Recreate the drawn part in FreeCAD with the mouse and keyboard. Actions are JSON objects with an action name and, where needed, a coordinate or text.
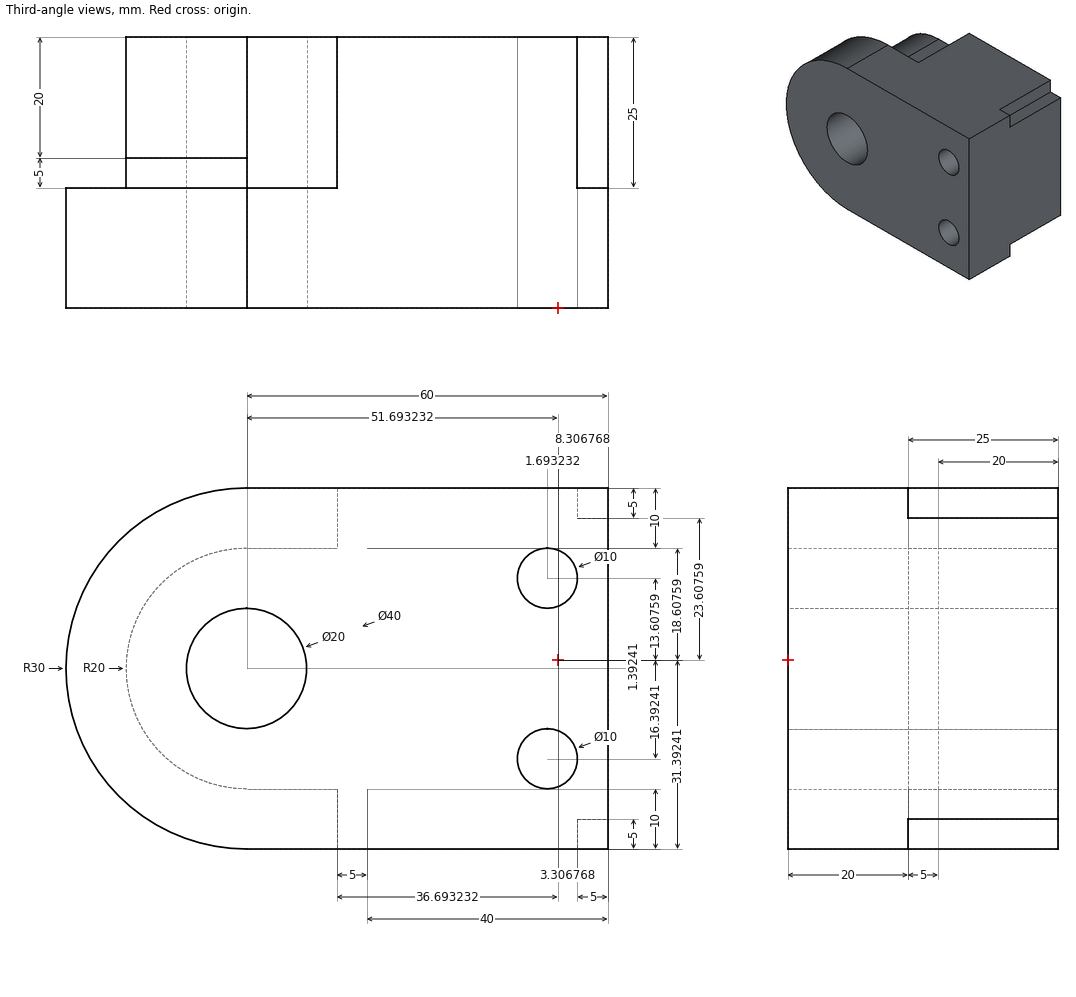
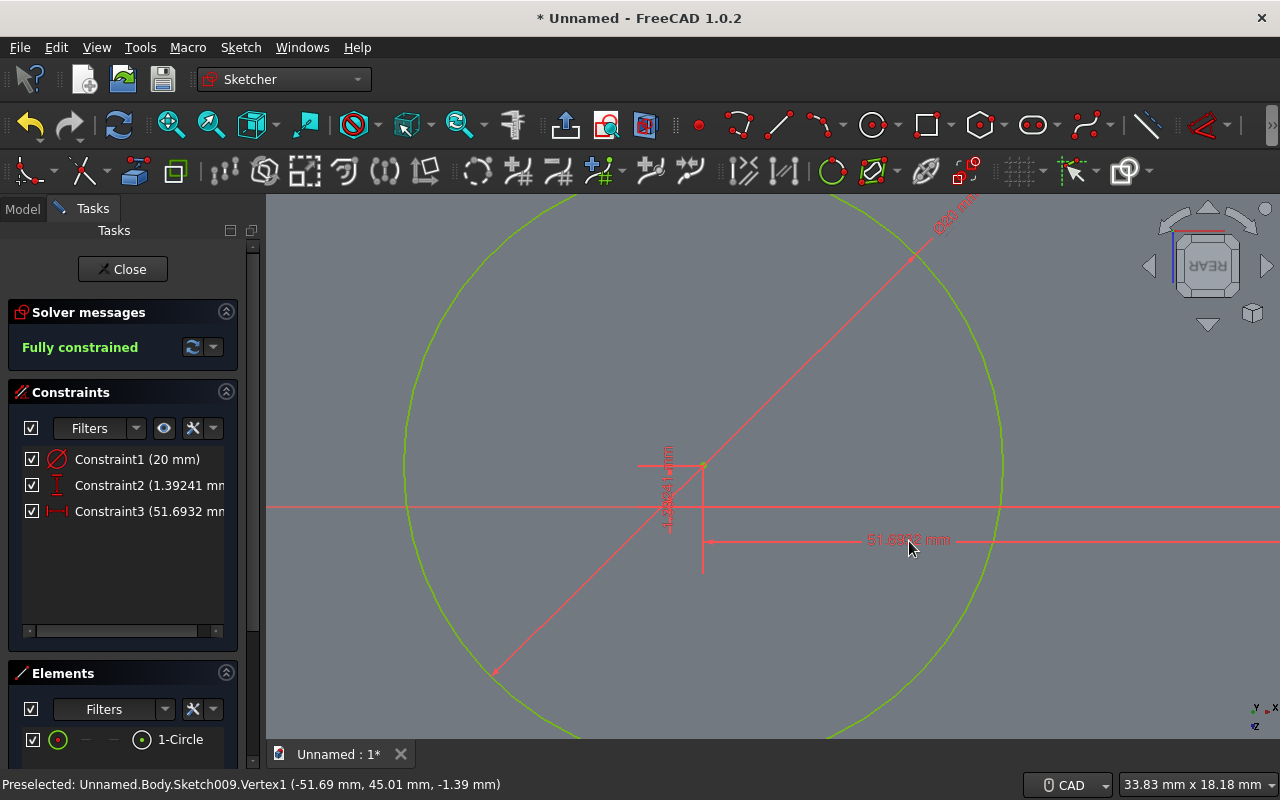
{"action": "left_click", "coordinate": [123, 269]}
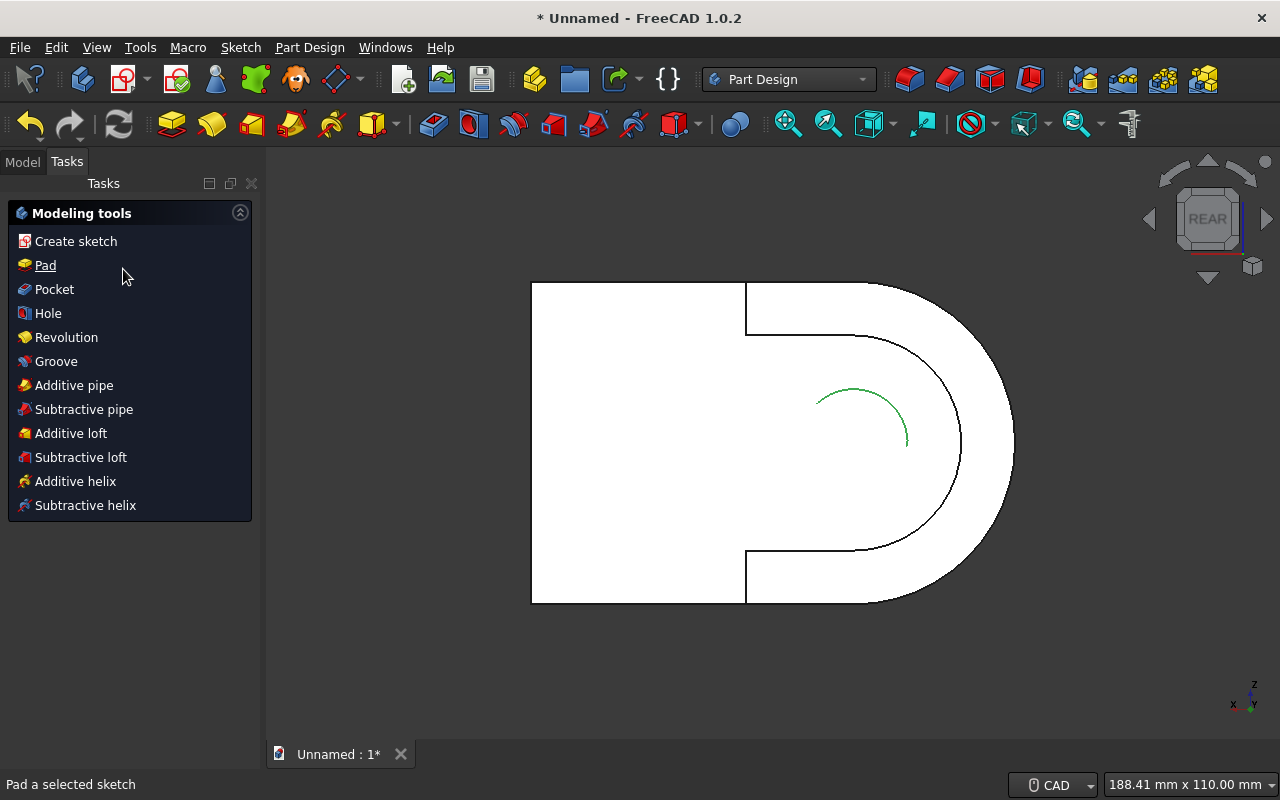
{"action": "left_click", "coordinate": [434, 124]}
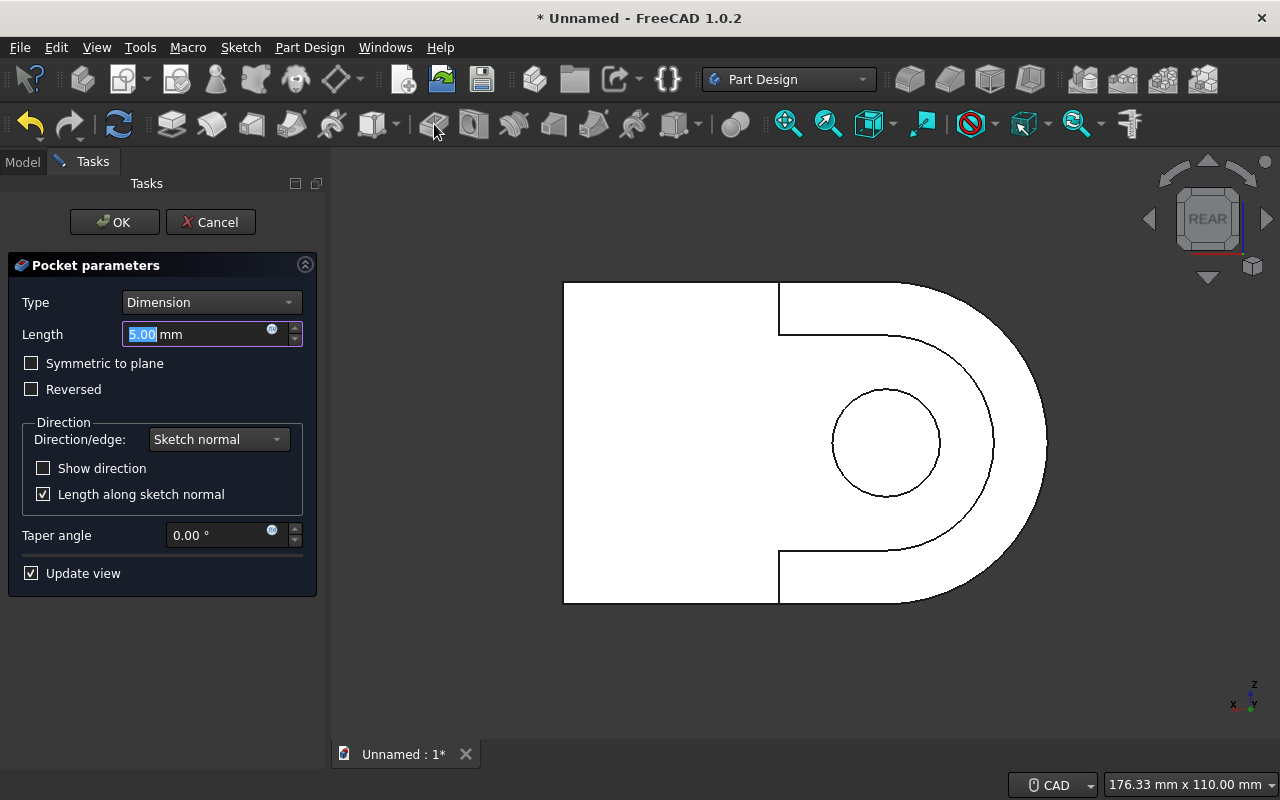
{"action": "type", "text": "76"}
{"action": "key", "text": "Tab"}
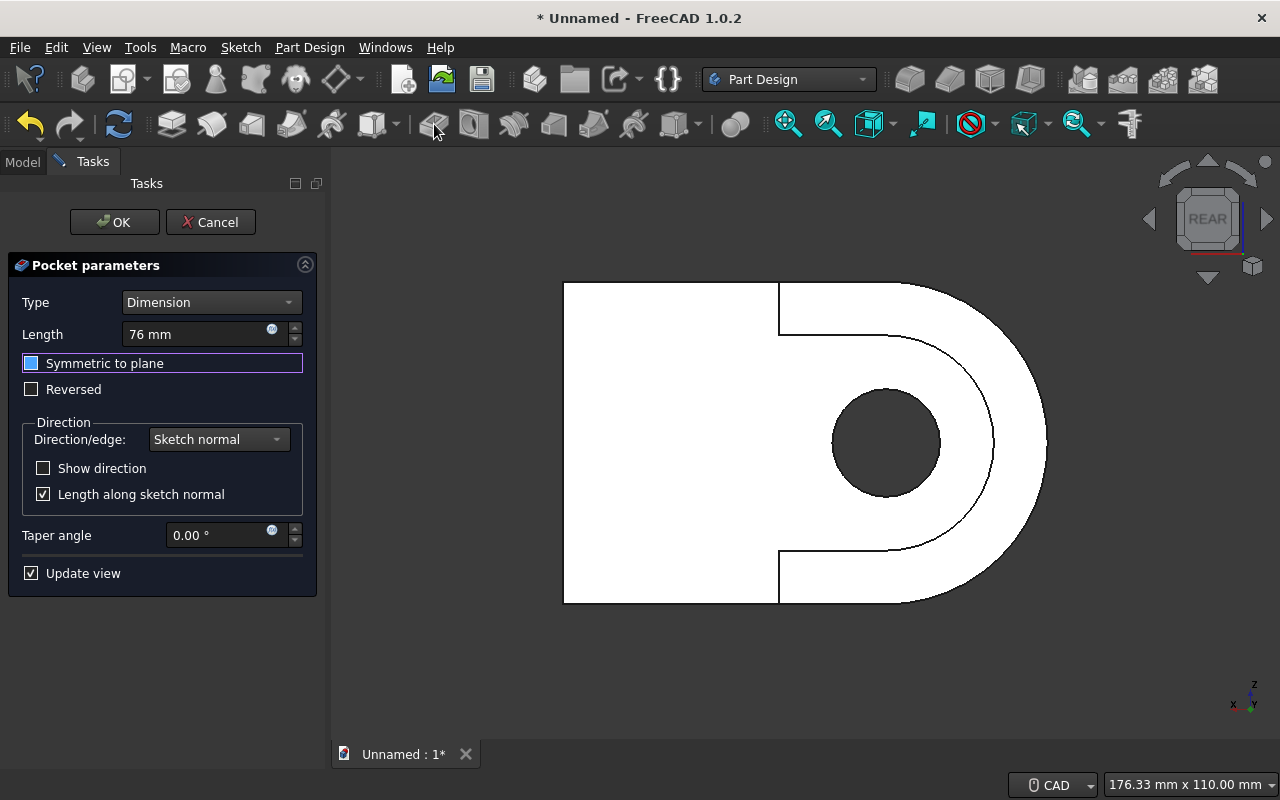
{"action": "left_click", "coordinate": [115, 222]}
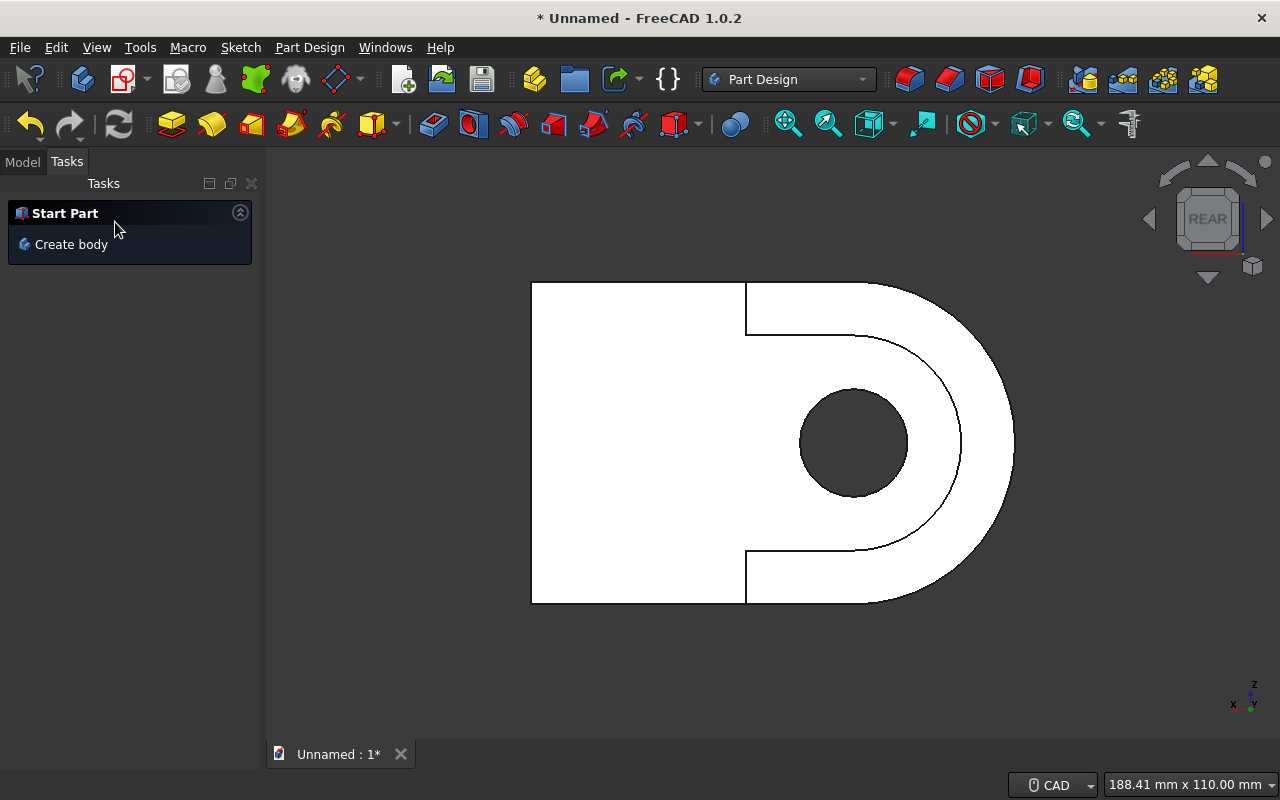
{"action": "left_click", "coordinate": [685, 442]}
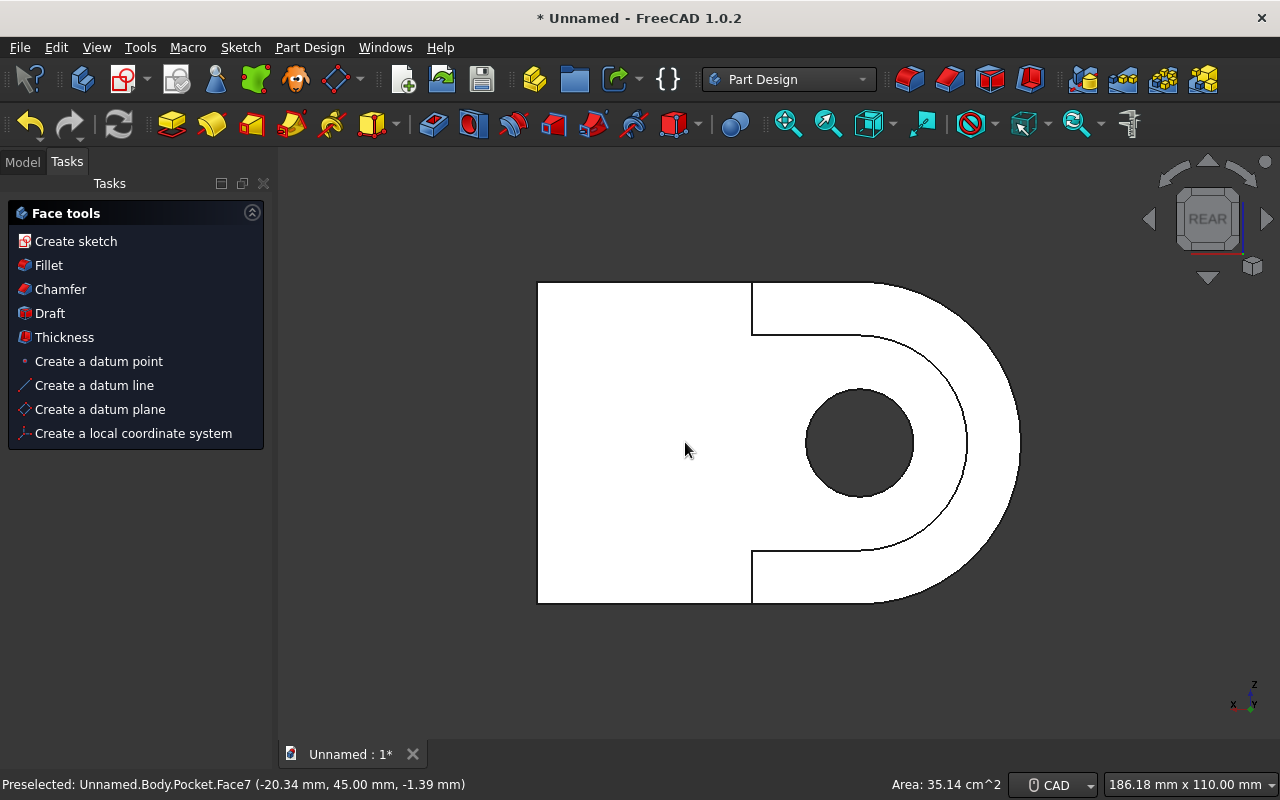
{"action": "left_click", "coordinate": [124, 80]}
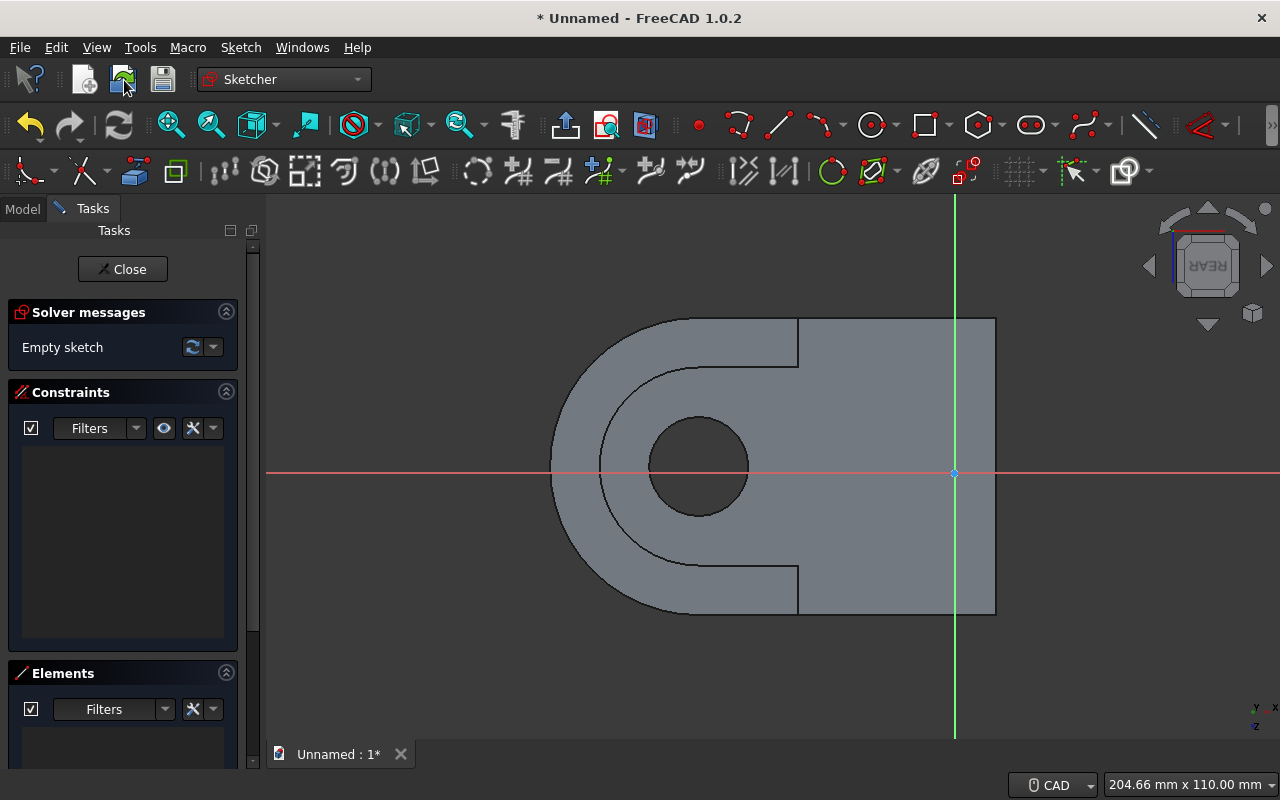
{"action": "scroll", "coordinate": [1006, 319], "scroll_direction": "up", "scroll_amount": 13}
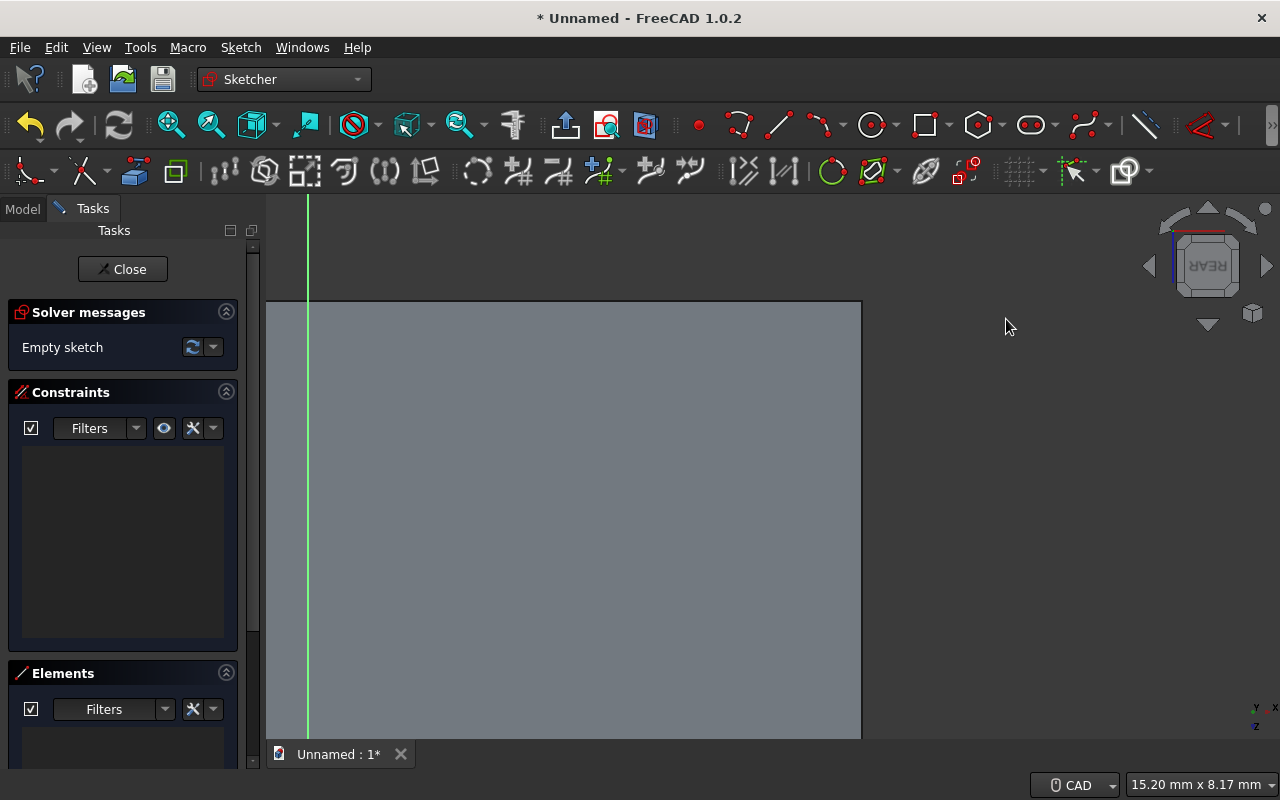
{"action": "key", "text": "g r"}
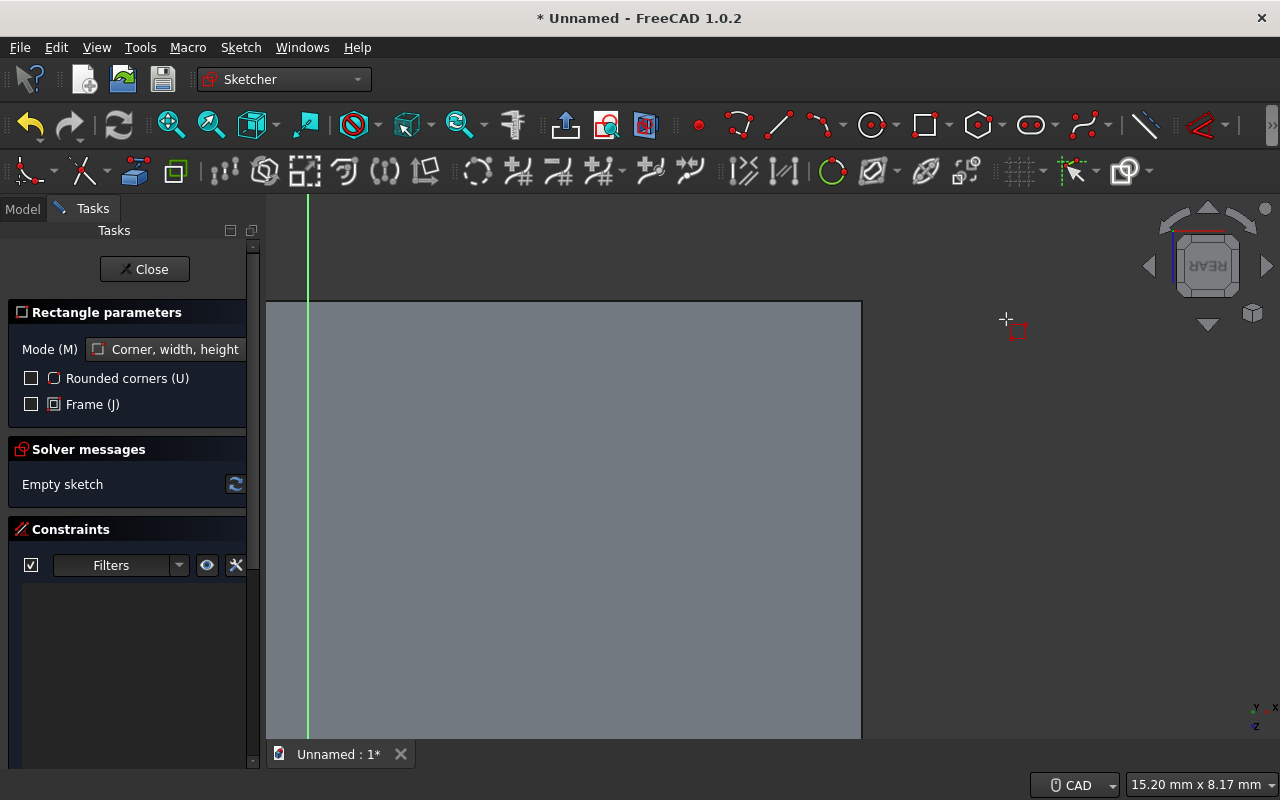
{"action": "left_click", "coordinate": [528, 301]}
{"action": "left_click", "coordinate": [862, 634]}
{"action": "key", "text": "Escape"}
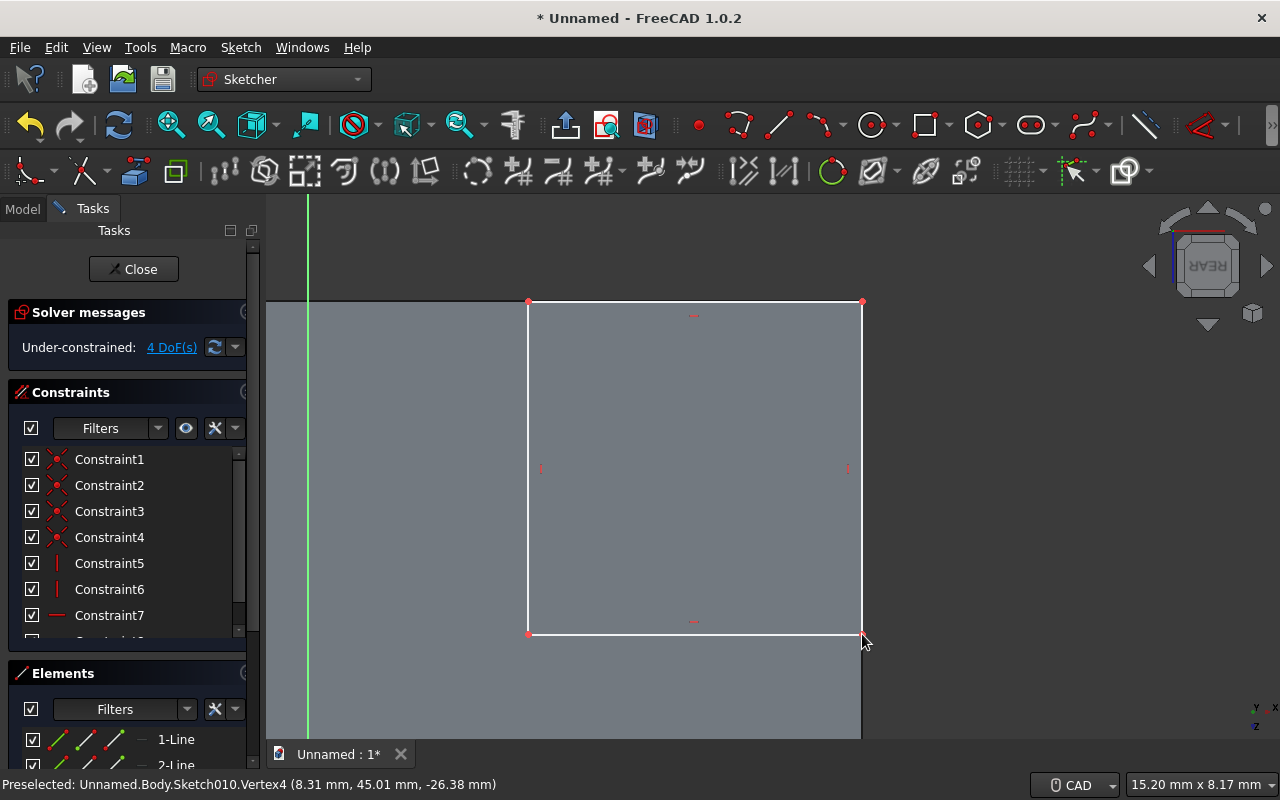
{"action": "key", "text": "d"}